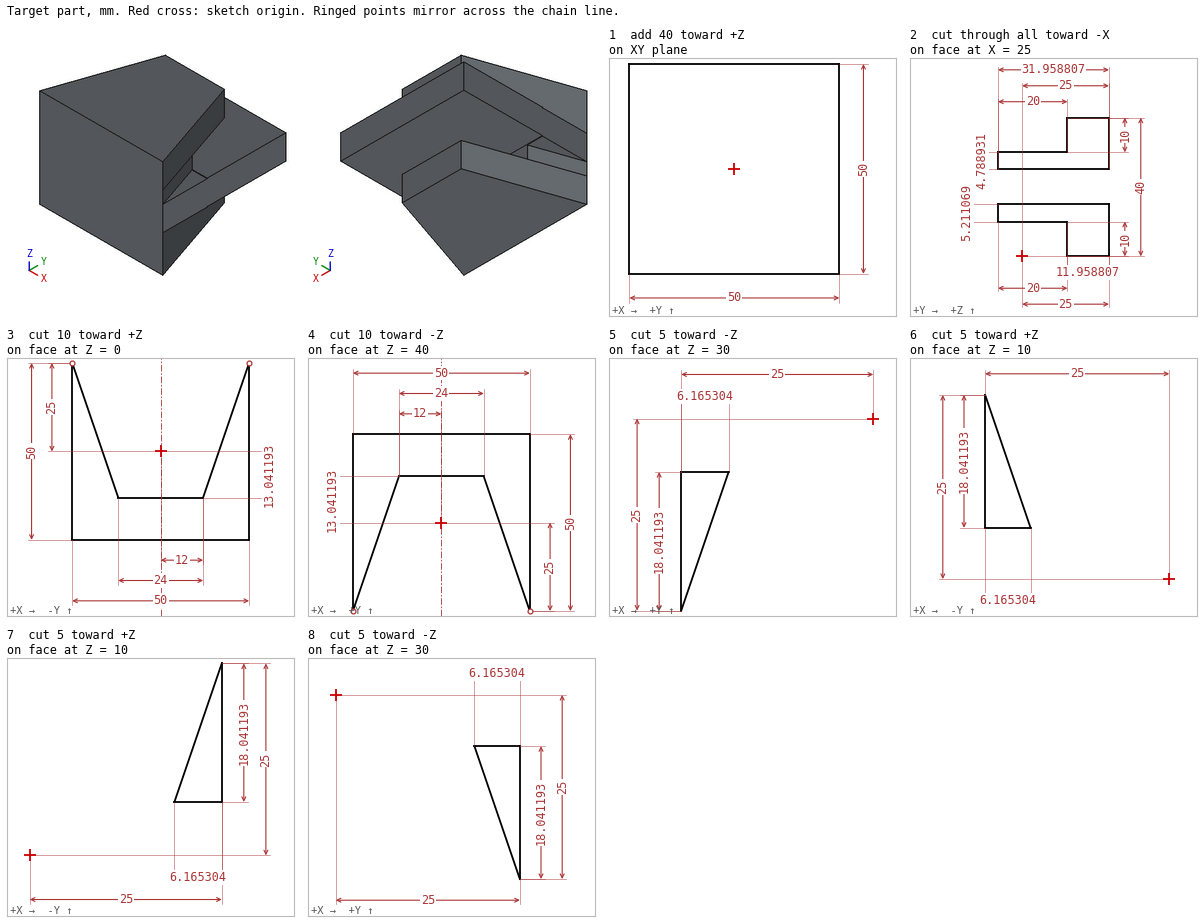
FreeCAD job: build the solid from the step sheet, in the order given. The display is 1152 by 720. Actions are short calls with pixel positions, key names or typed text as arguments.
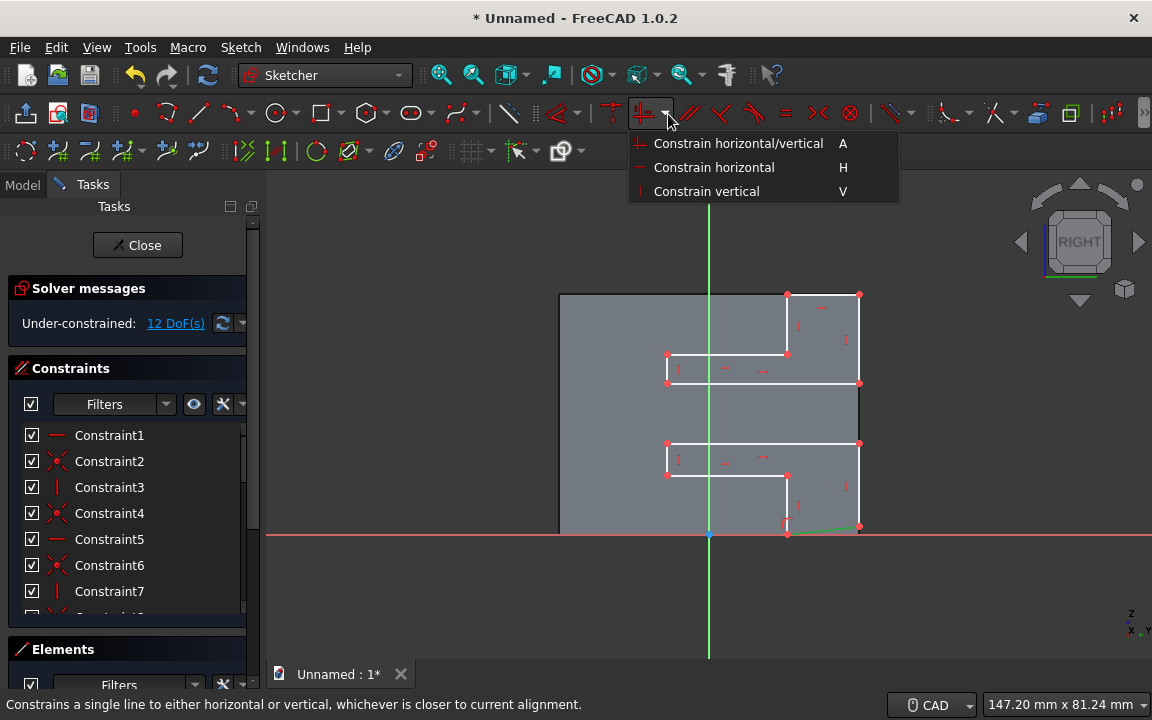
click(764, 167)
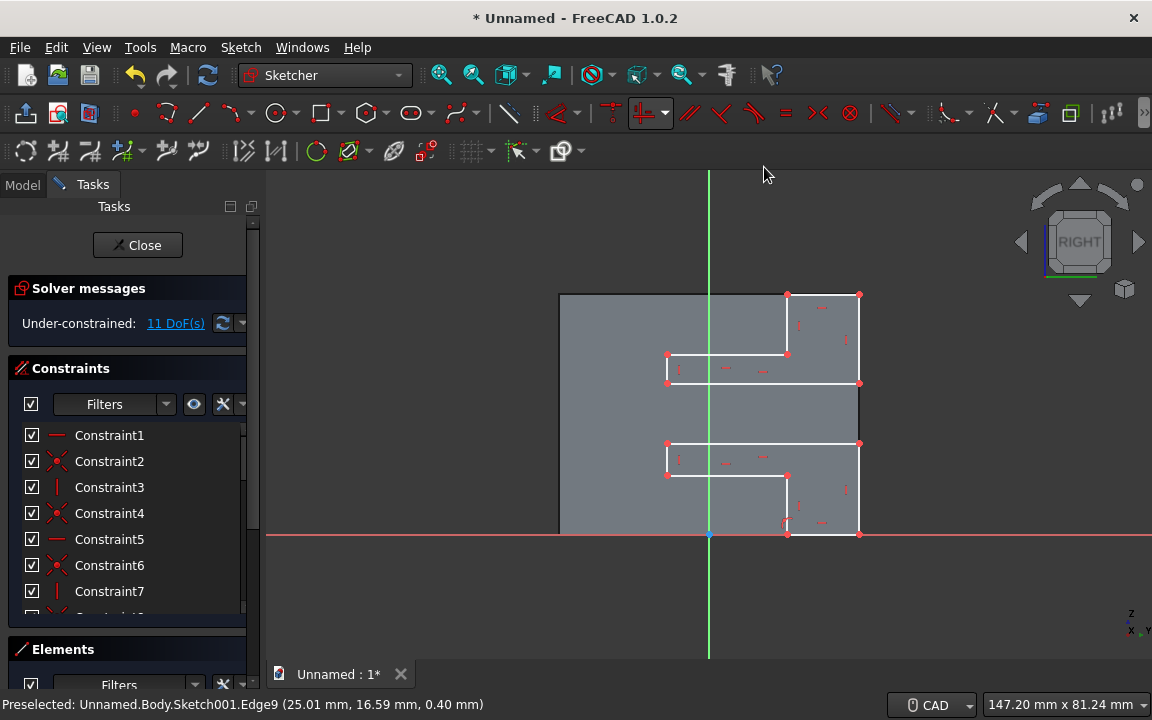
click(787, 313)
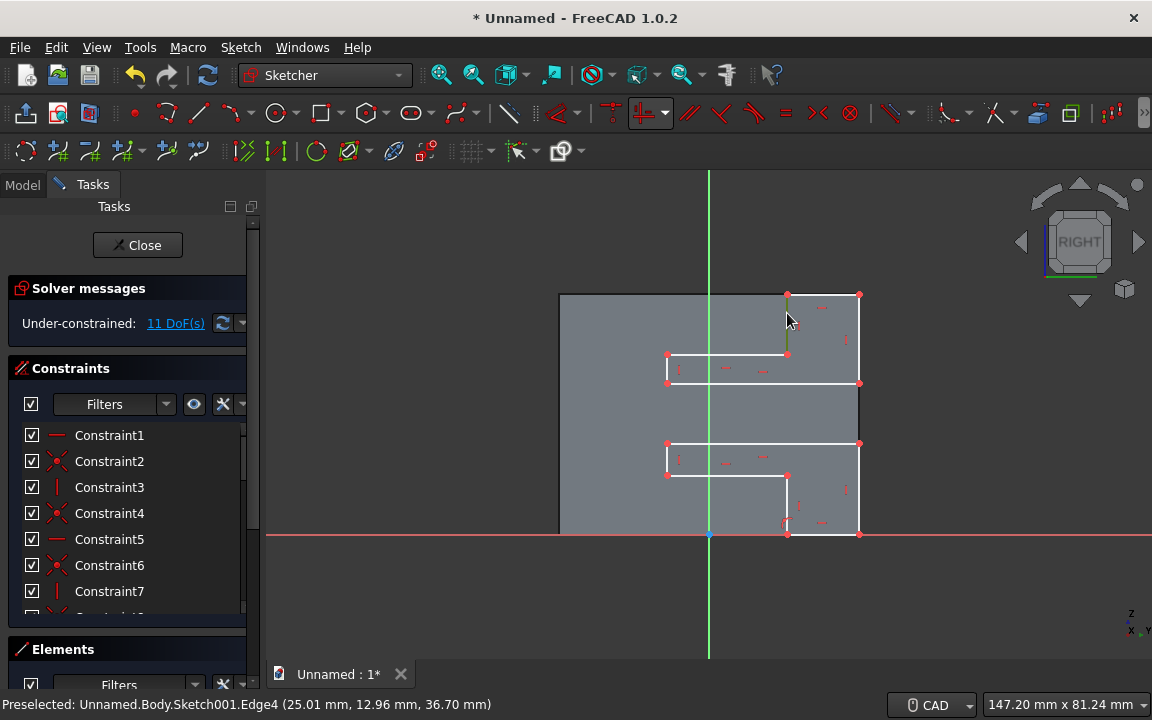
key(i)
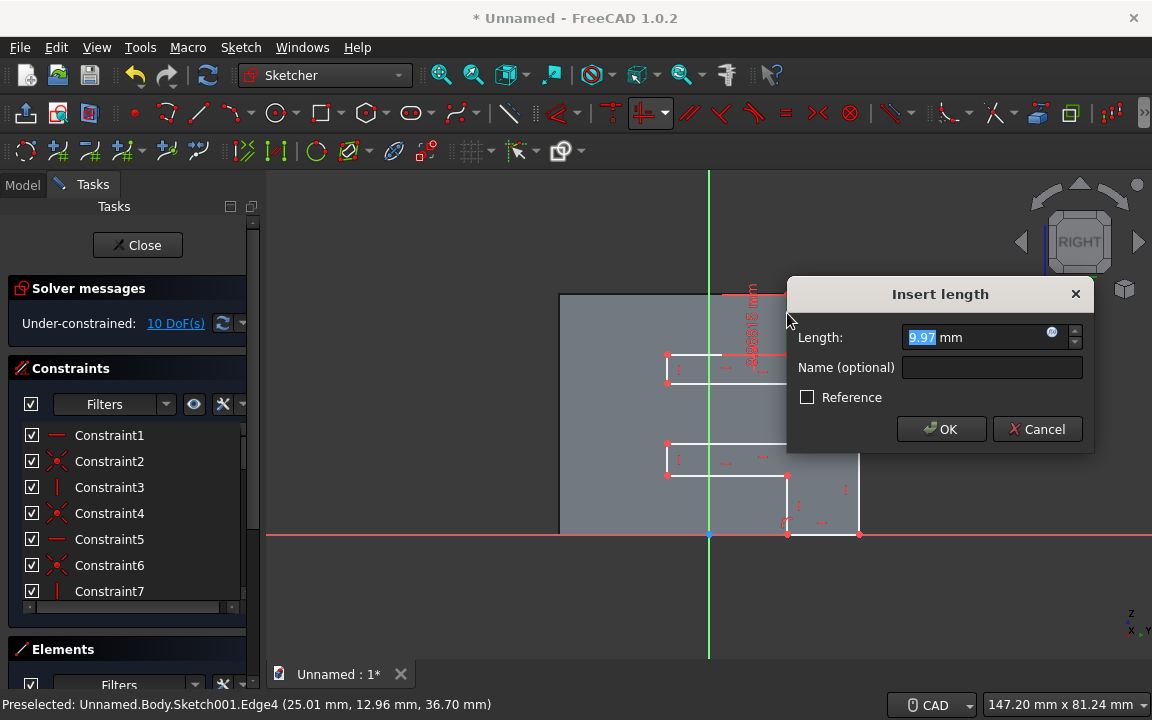
text(10)
key(Return)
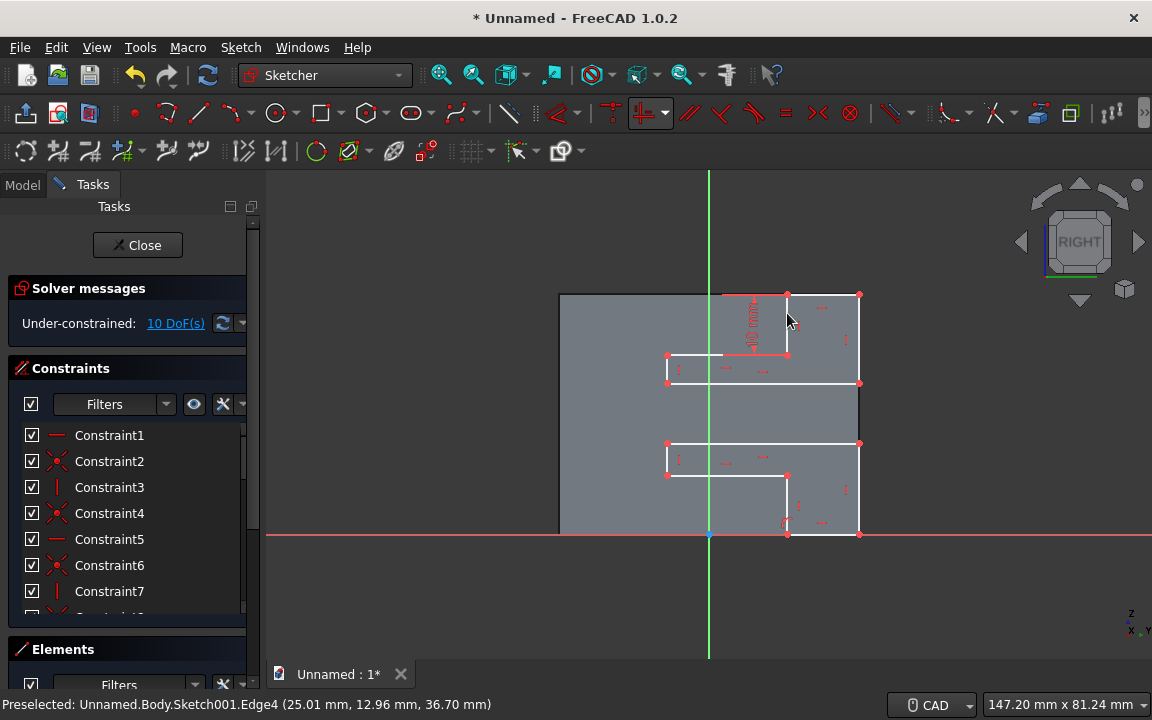
click(751, 355)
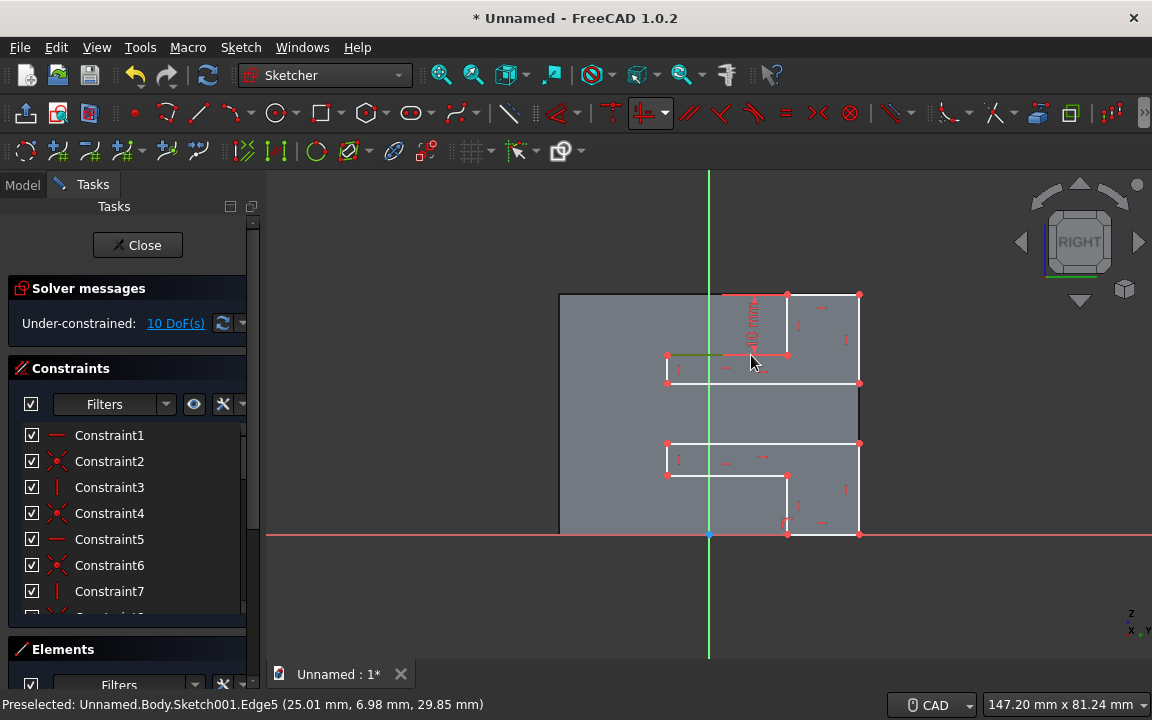
key(l)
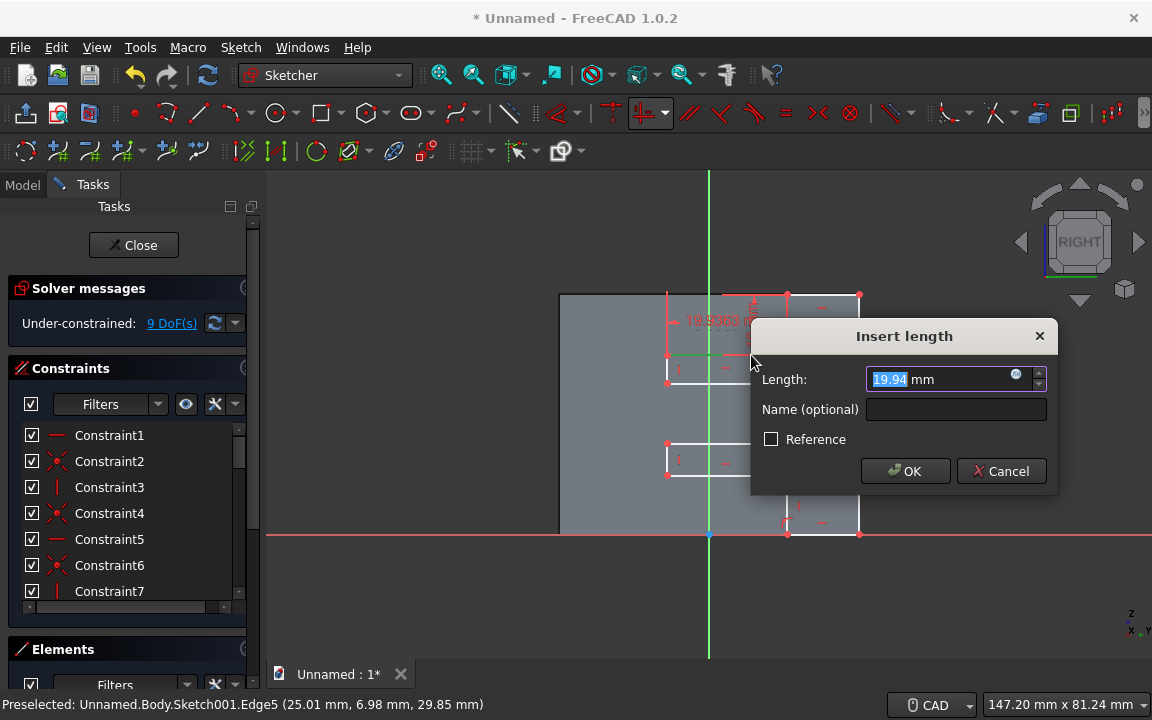
text(20)
key(Return)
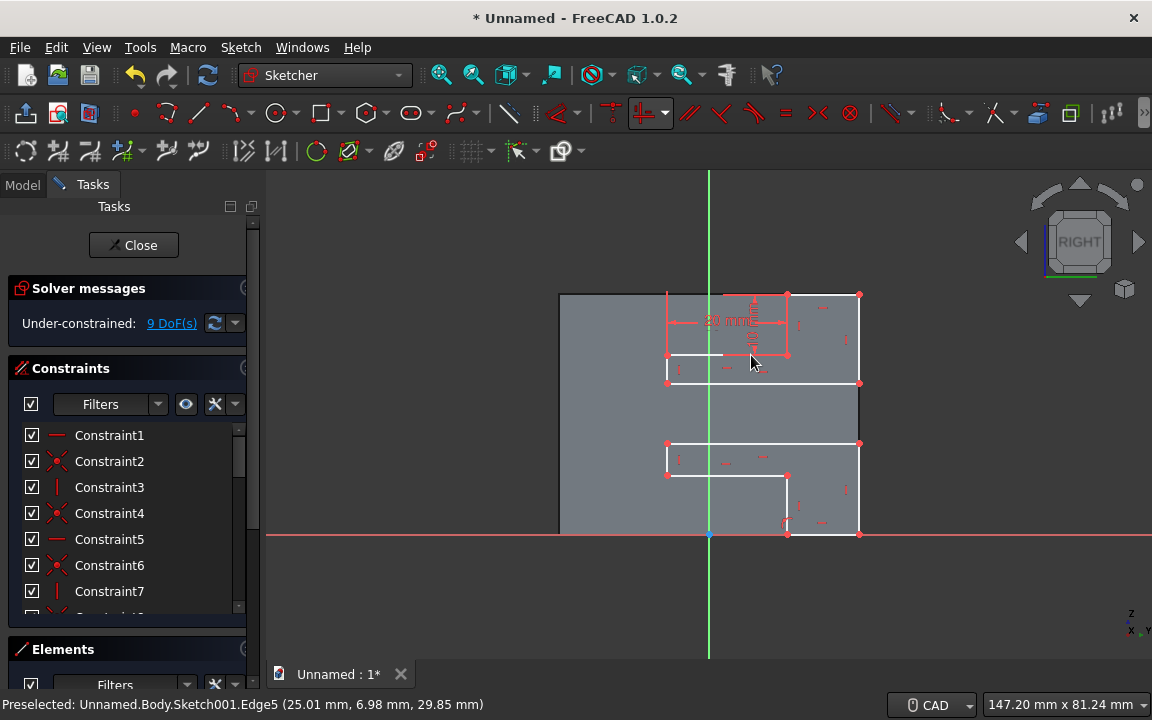
click(751, 476)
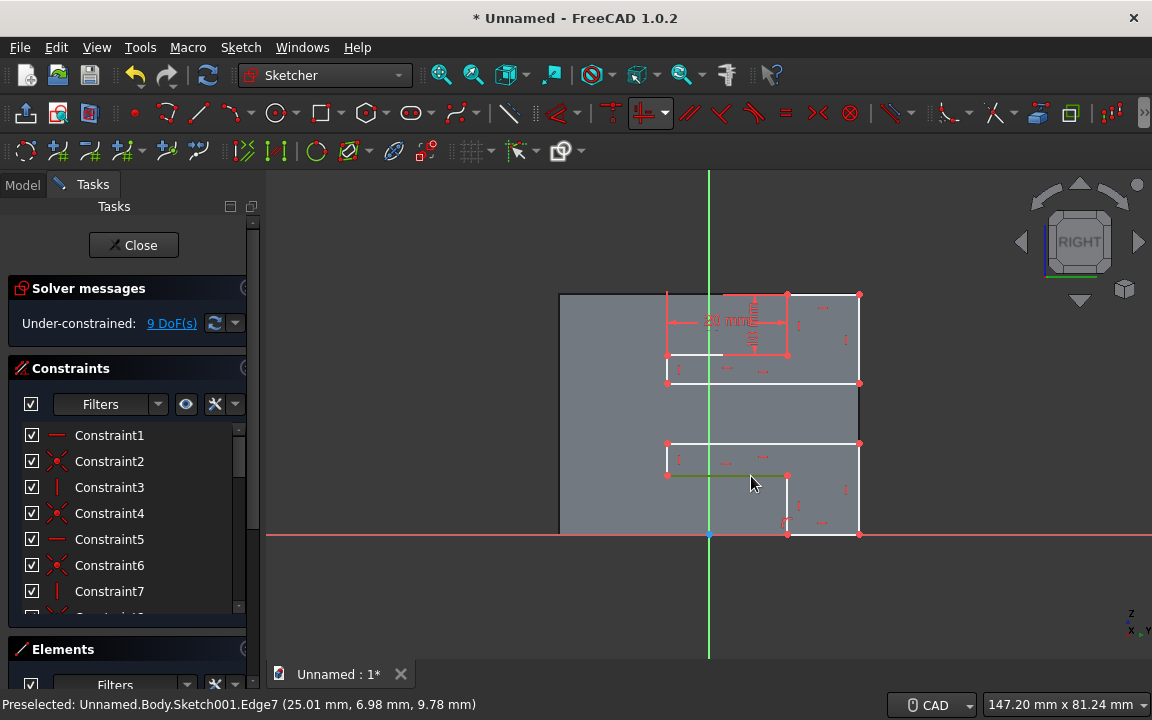
key(l)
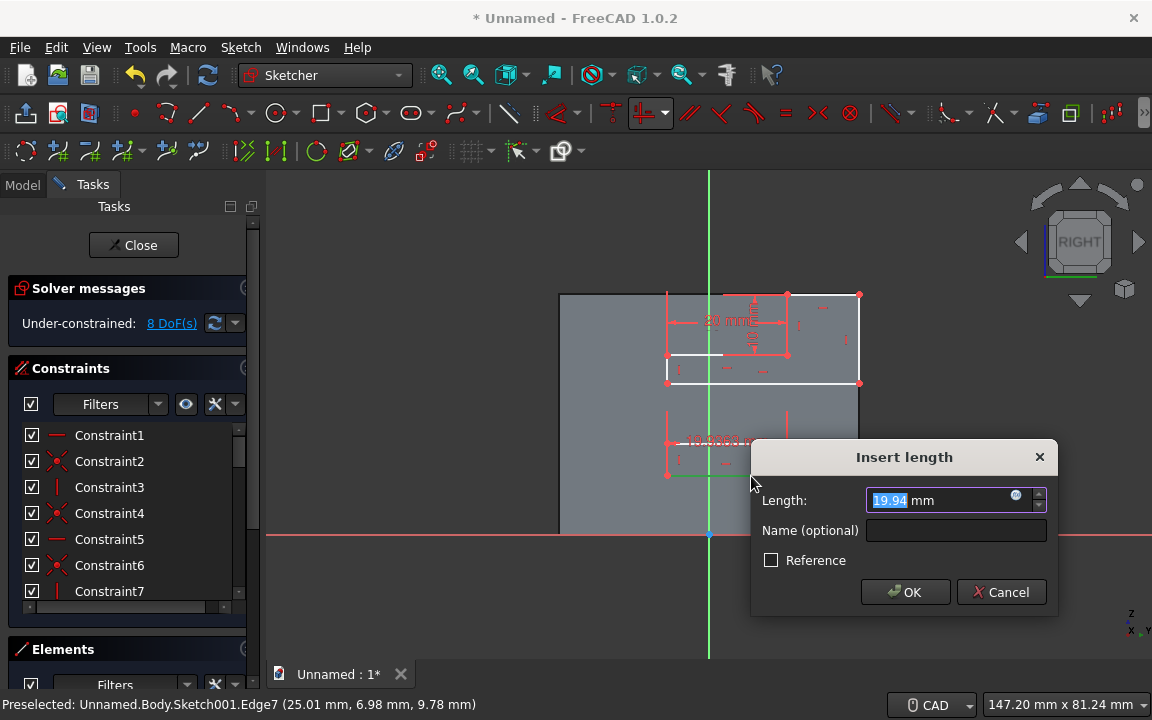
text(20)
key(Return)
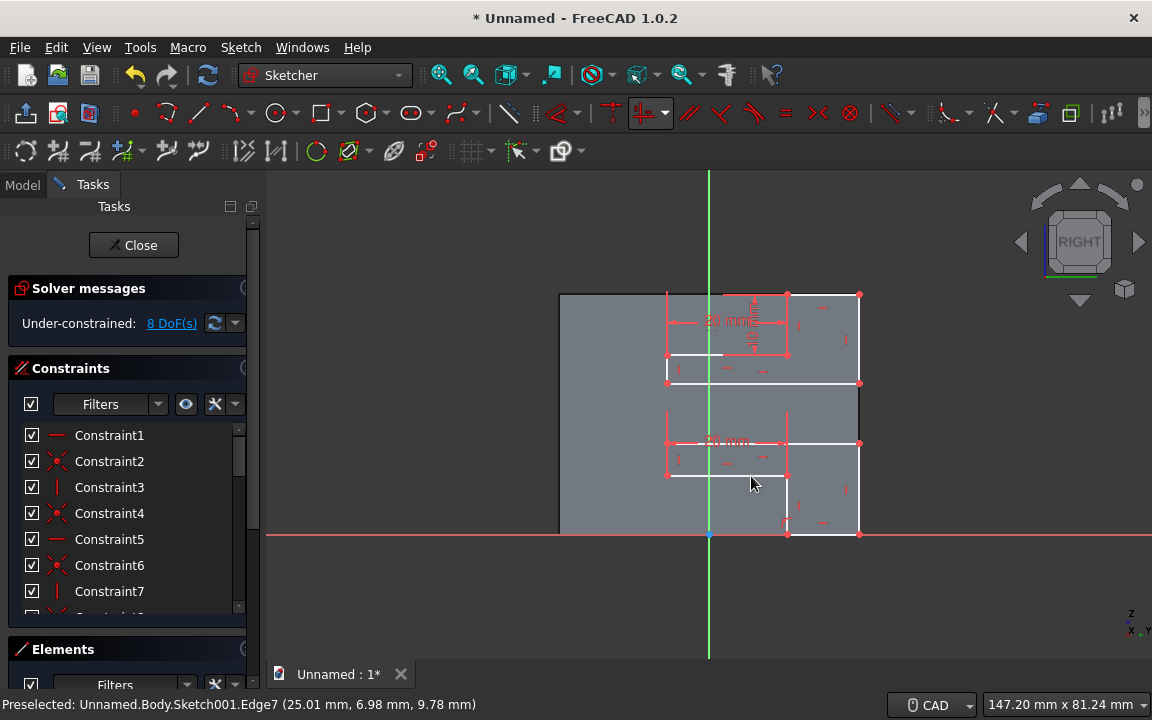
click(787, 494)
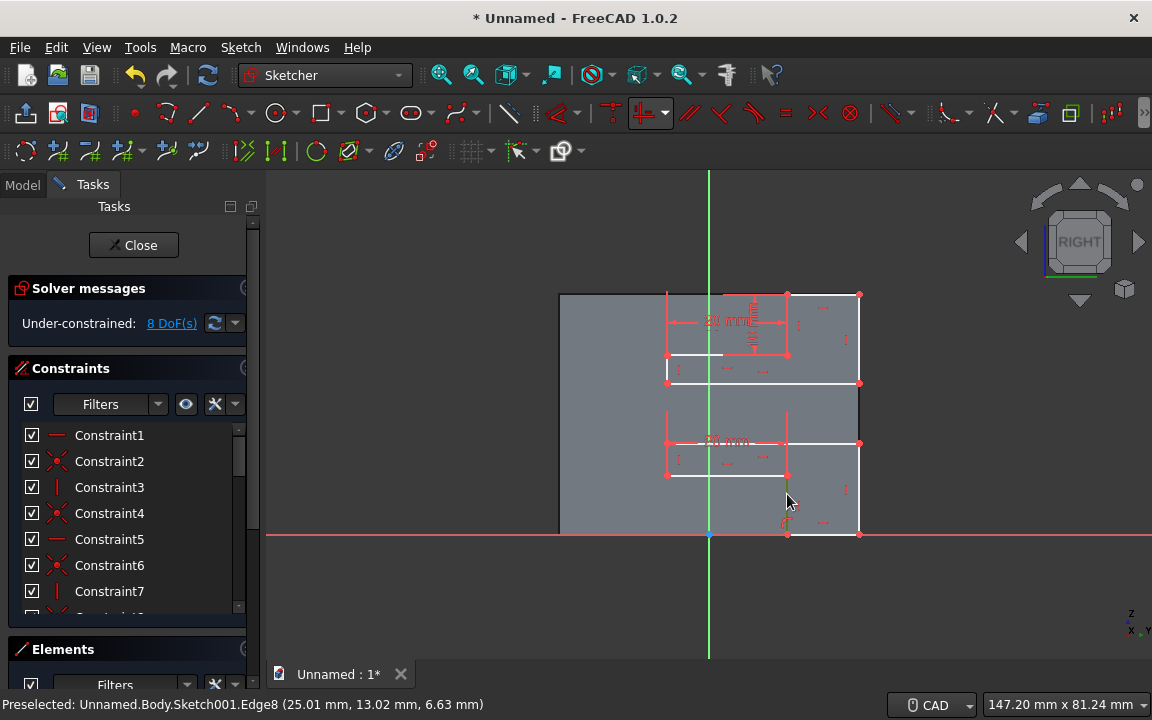
key(i)